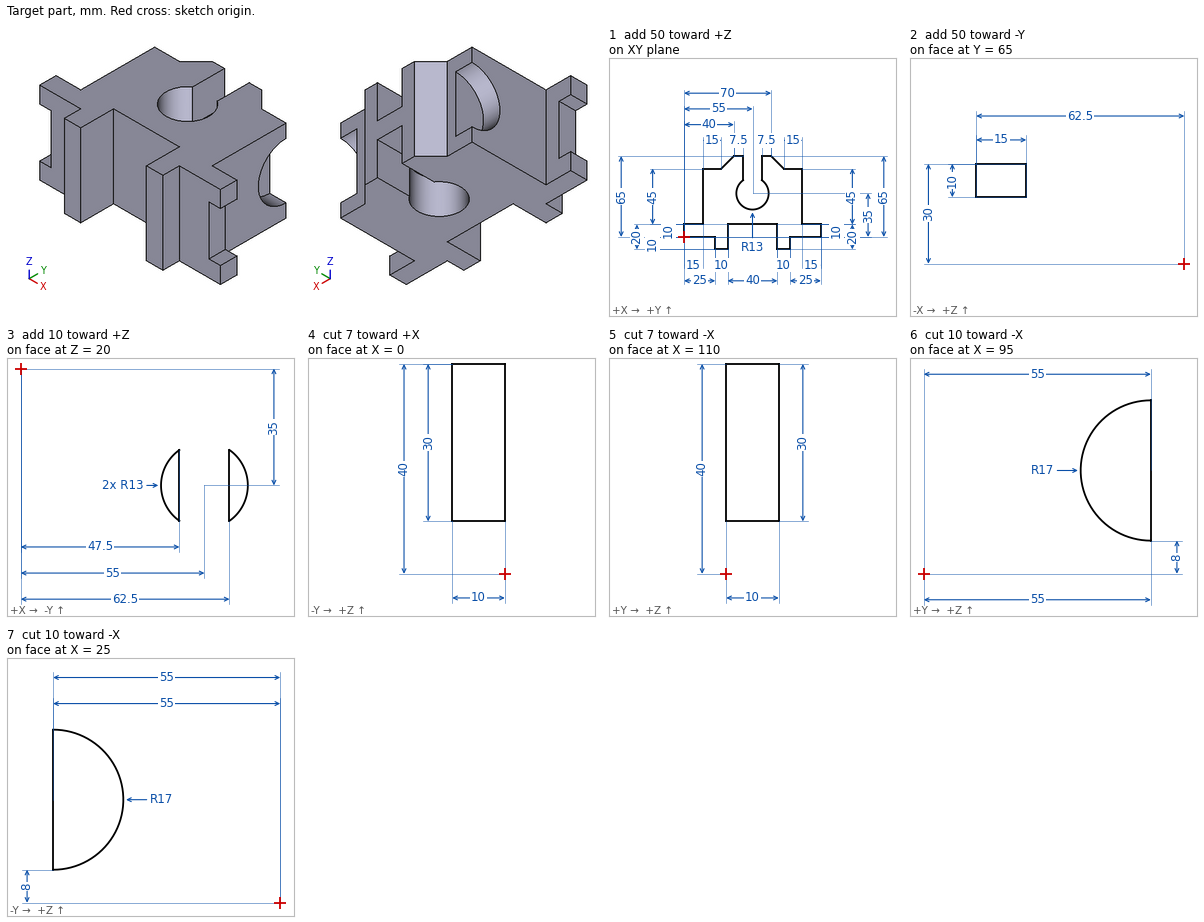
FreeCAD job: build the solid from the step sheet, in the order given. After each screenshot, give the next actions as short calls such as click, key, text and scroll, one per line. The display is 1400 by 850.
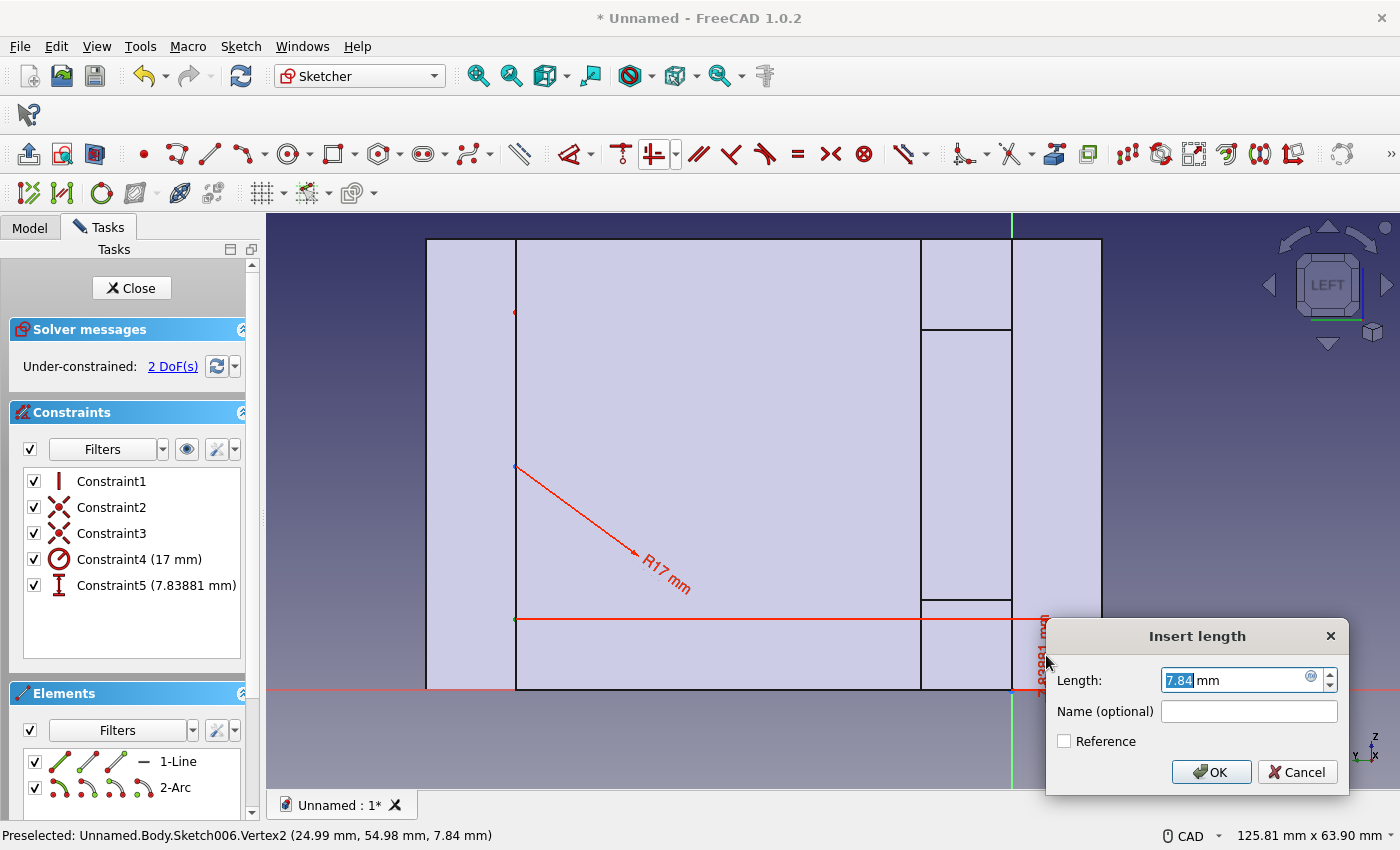
text(8)
key(Return)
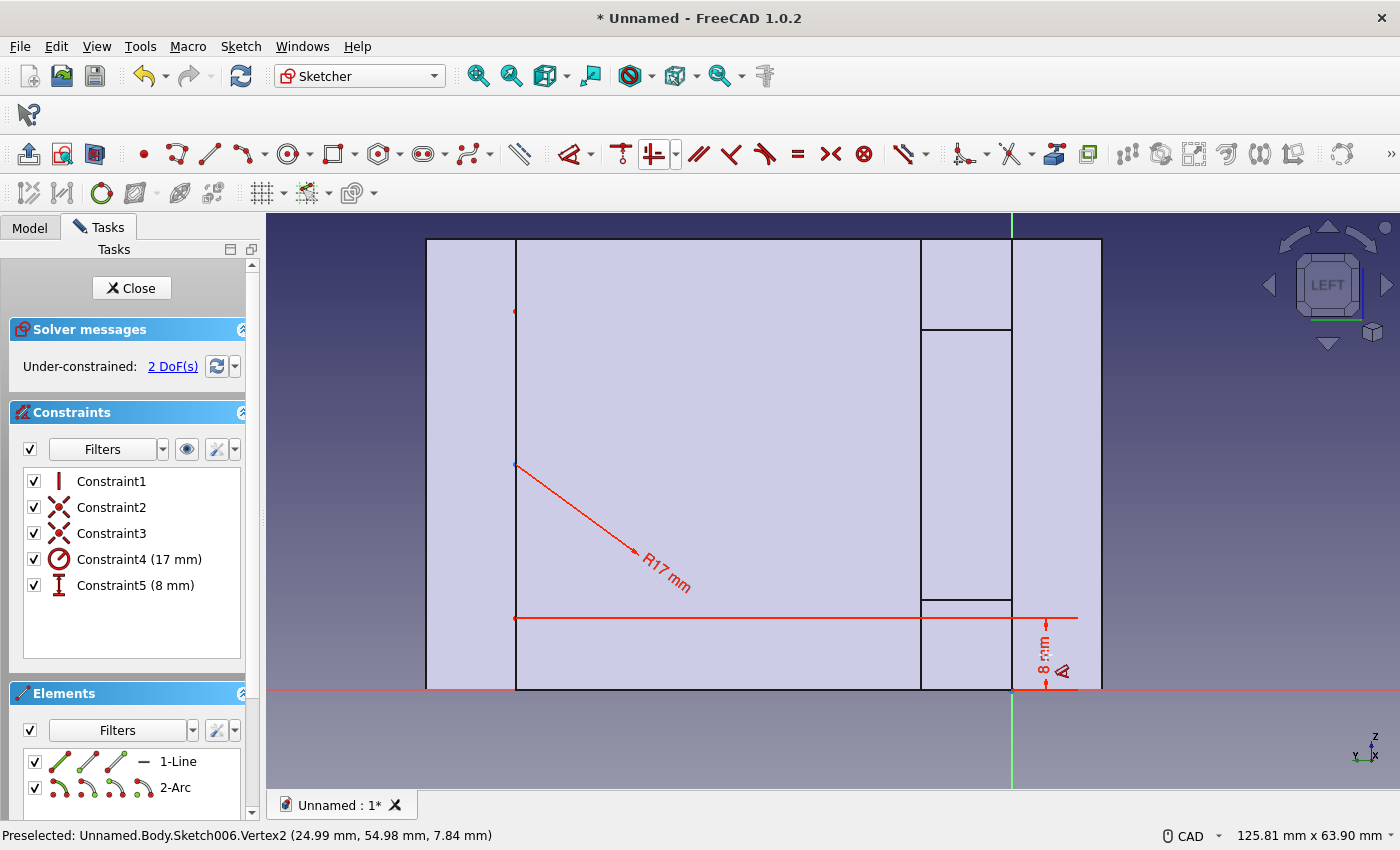
click(516, 312)
click(764, 724)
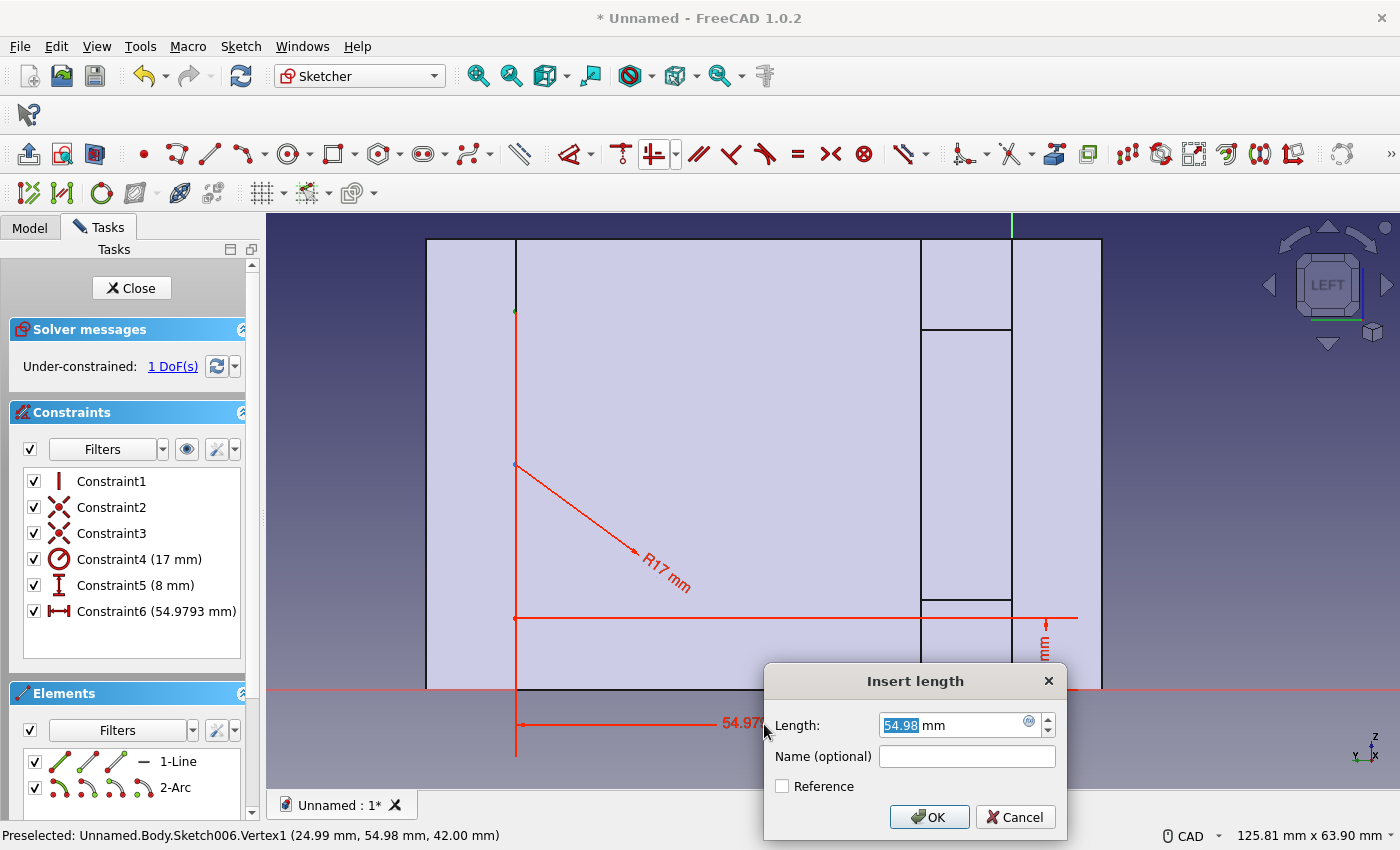
text(55)
key(Return)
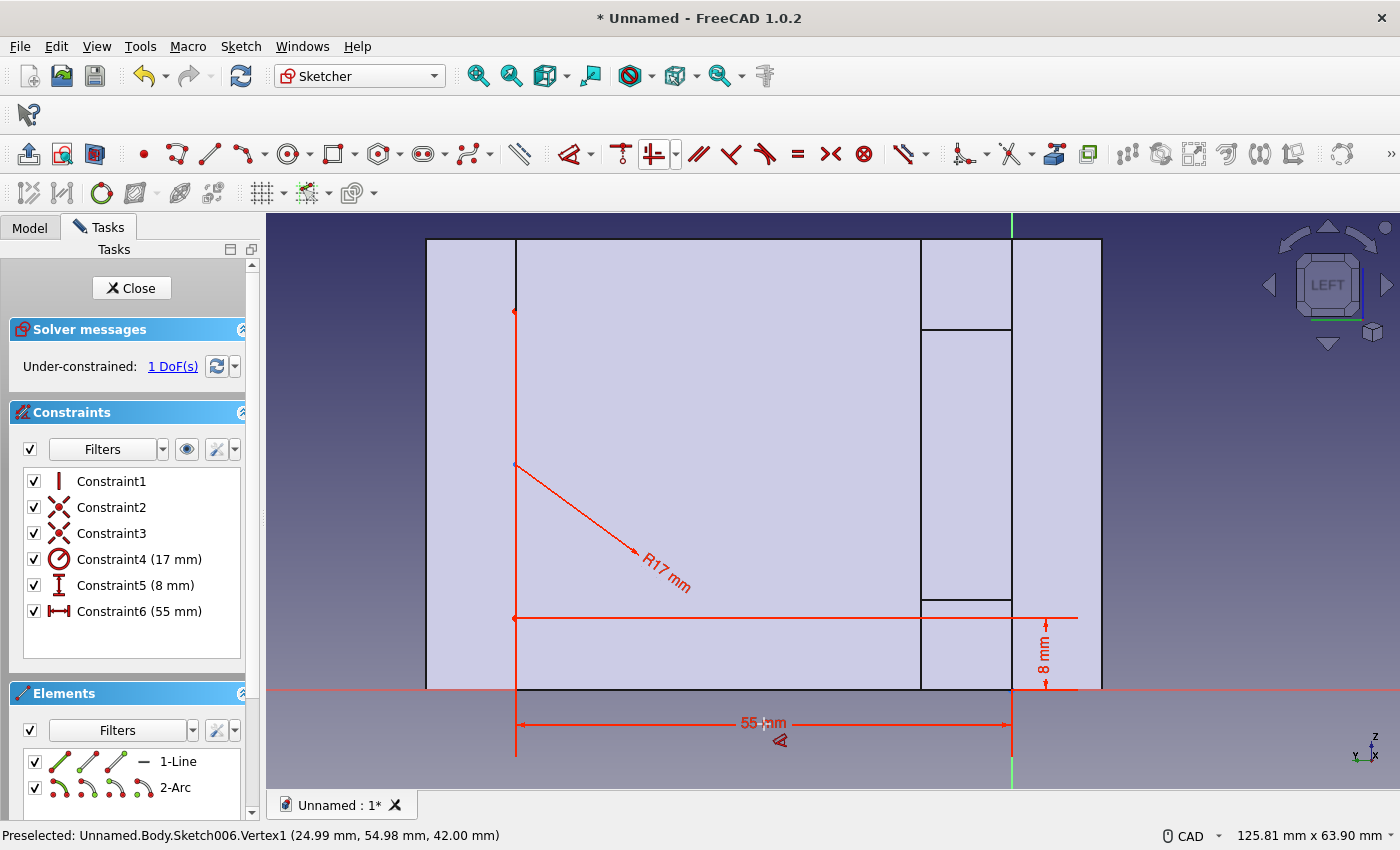
click(516, 465)
click(650, 724)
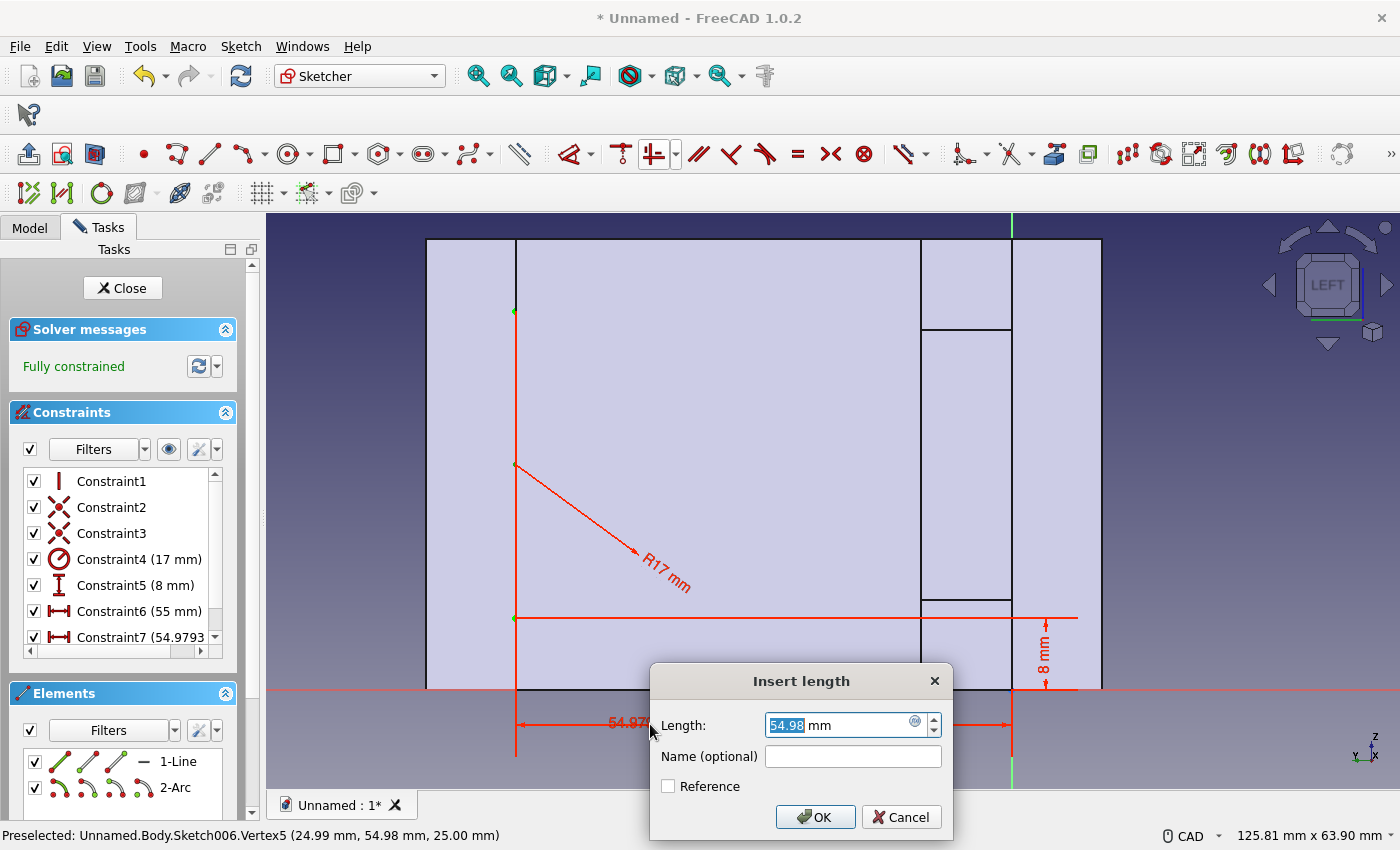
text(55)
key(Return)
key(Escape)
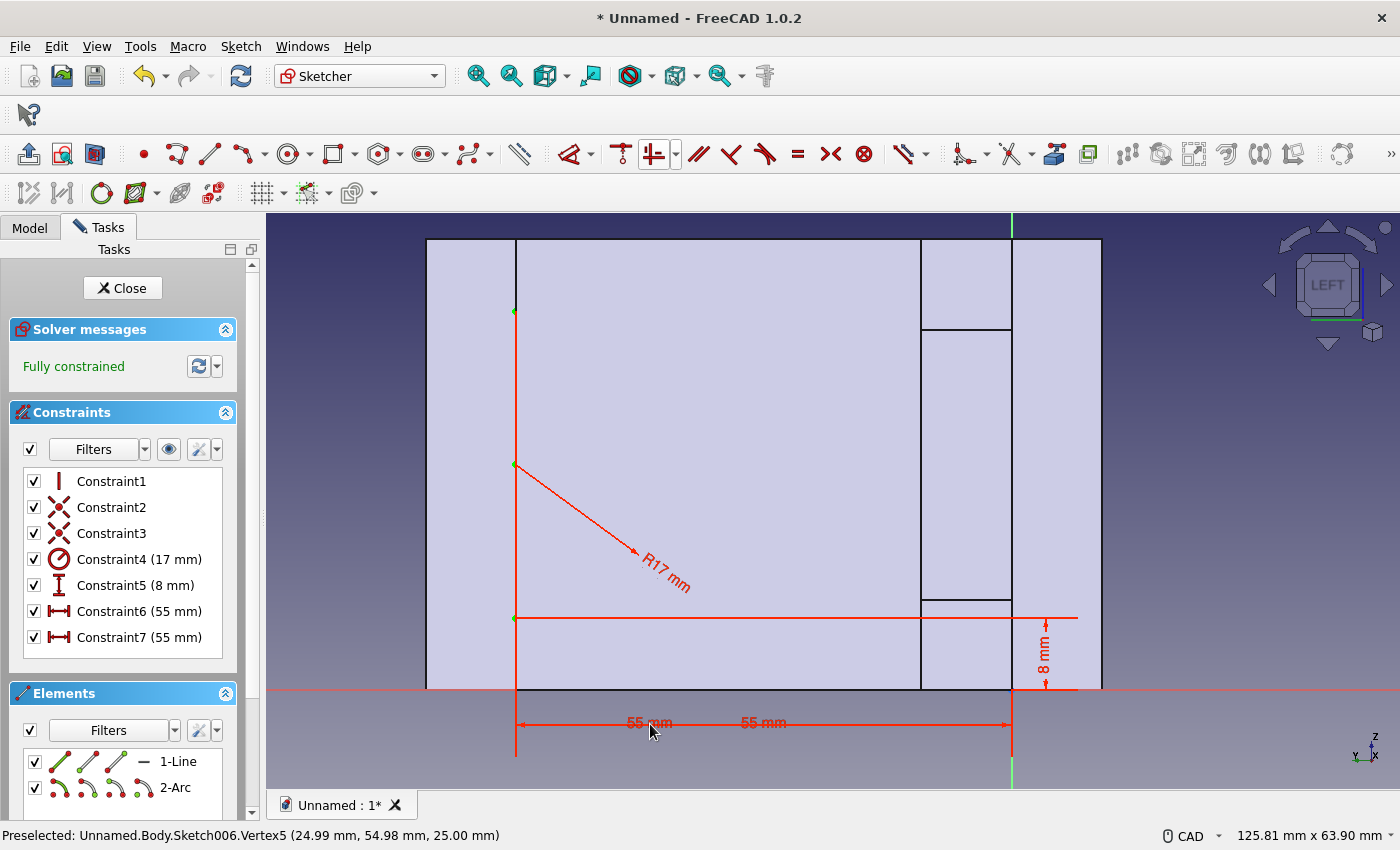
click(123, 288)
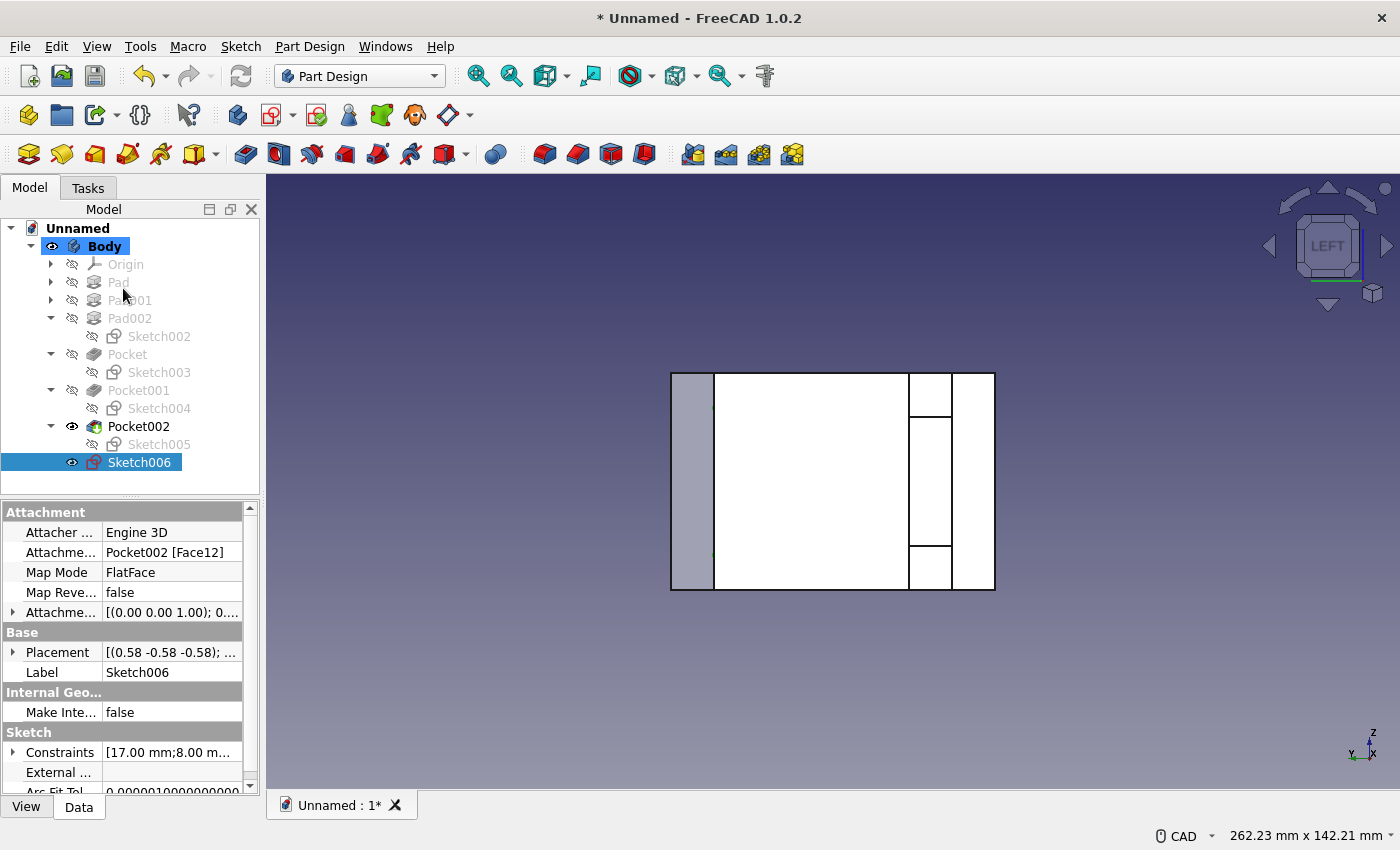
click(246, 154)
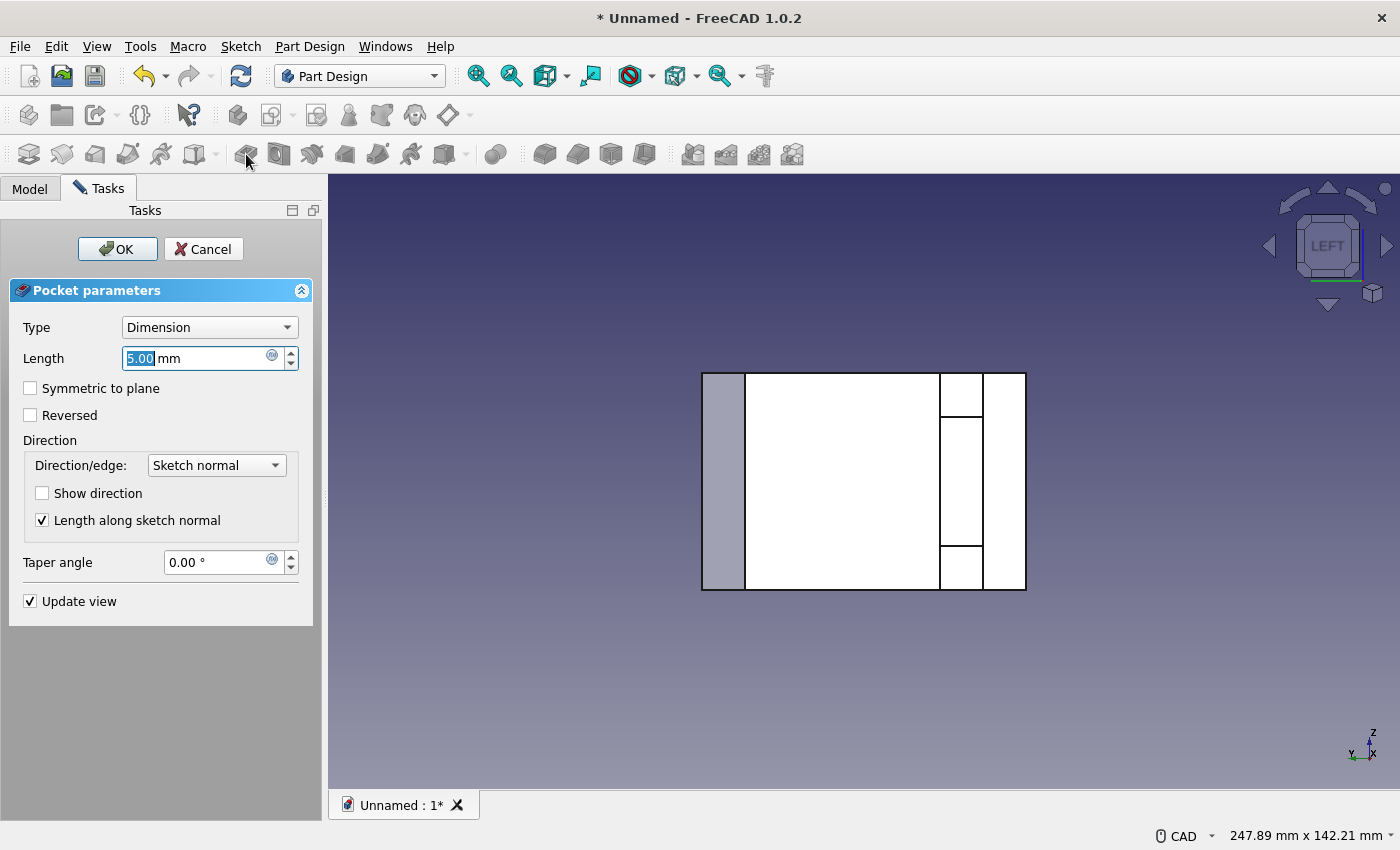
text(10)
key(Tab)